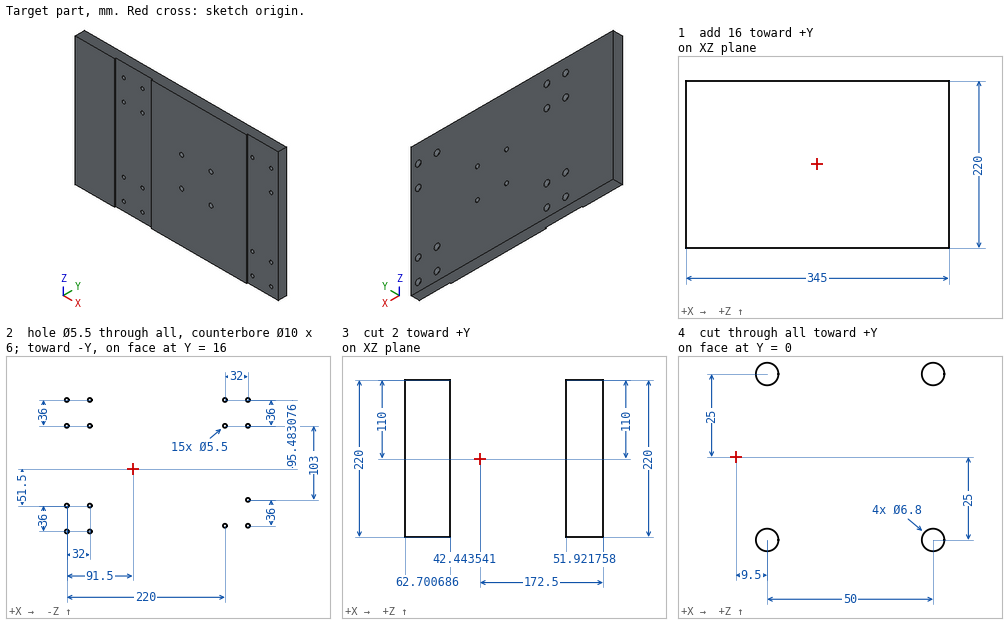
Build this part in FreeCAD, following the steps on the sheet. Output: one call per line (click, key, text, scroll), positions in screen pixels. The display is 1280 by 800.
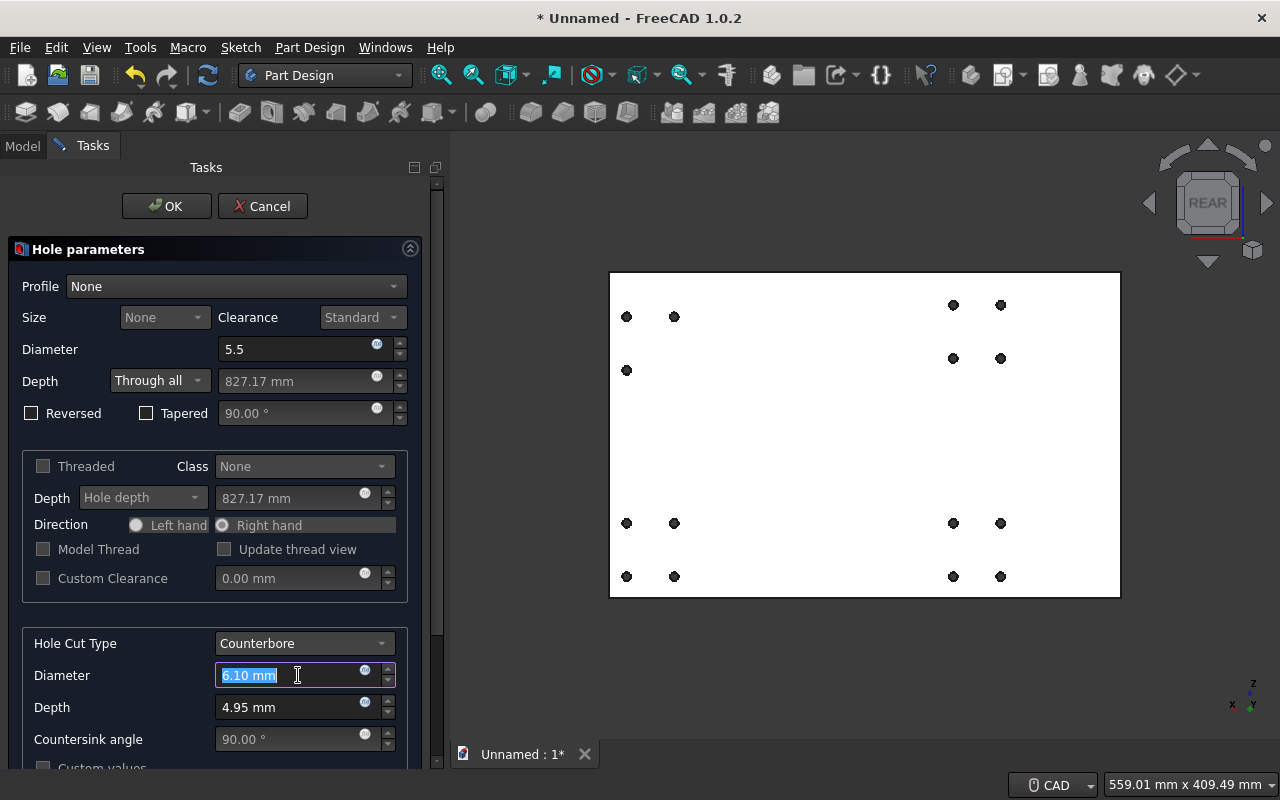
text(10)
key(Tab)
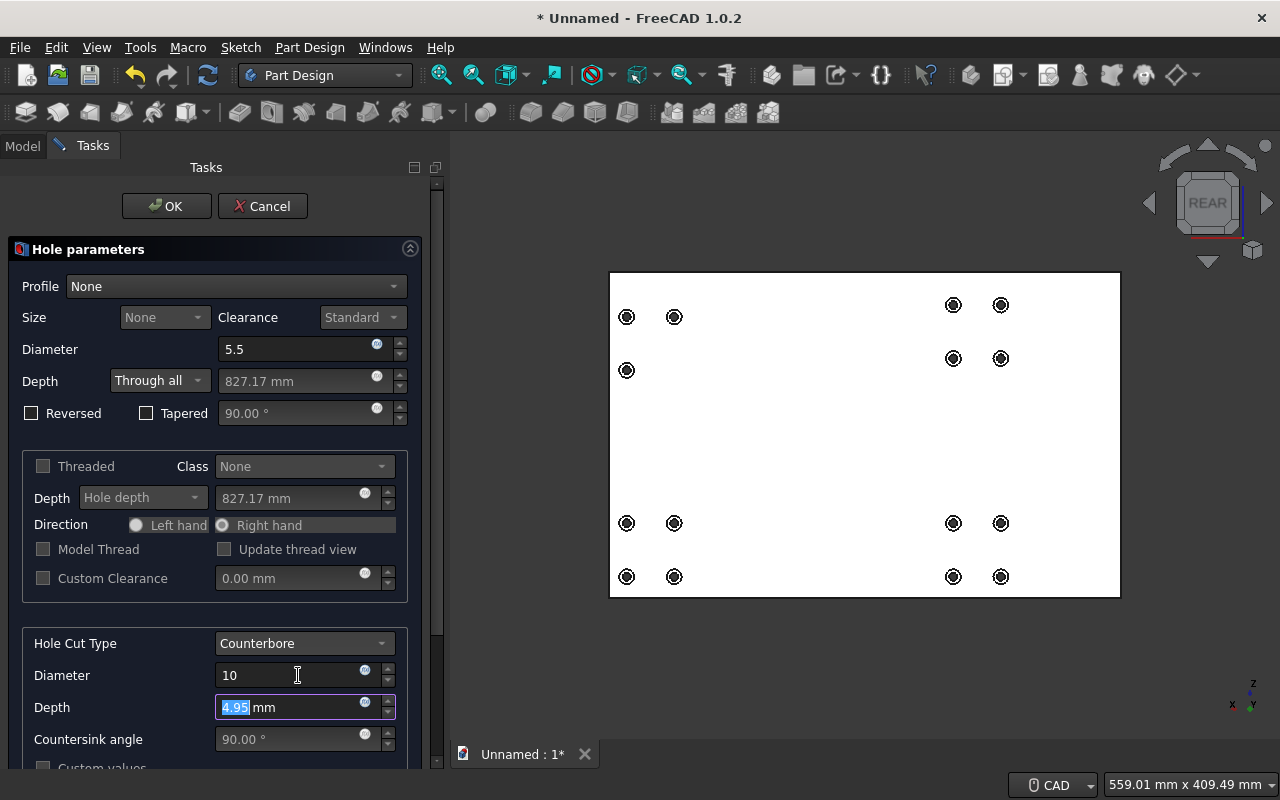
text(6)
key(Tab)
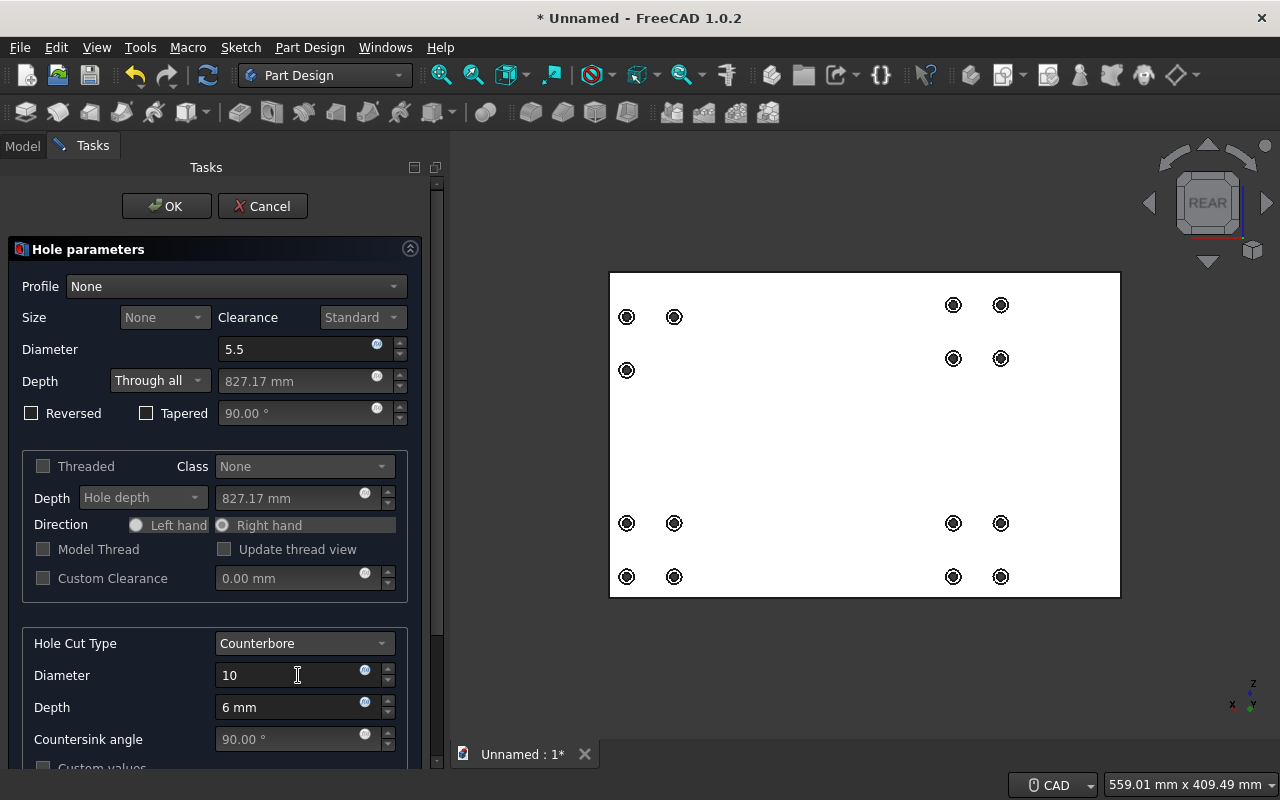
click(167, 206)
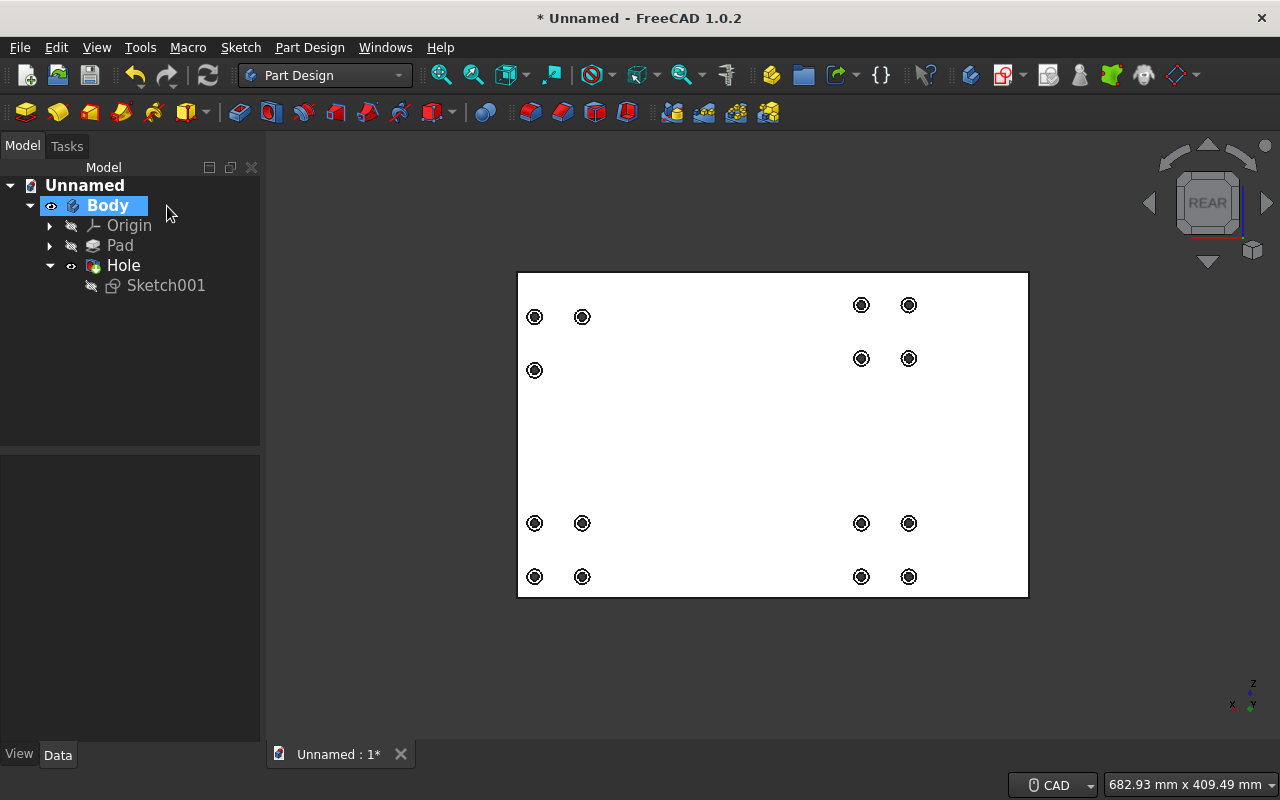
click(1004, 76)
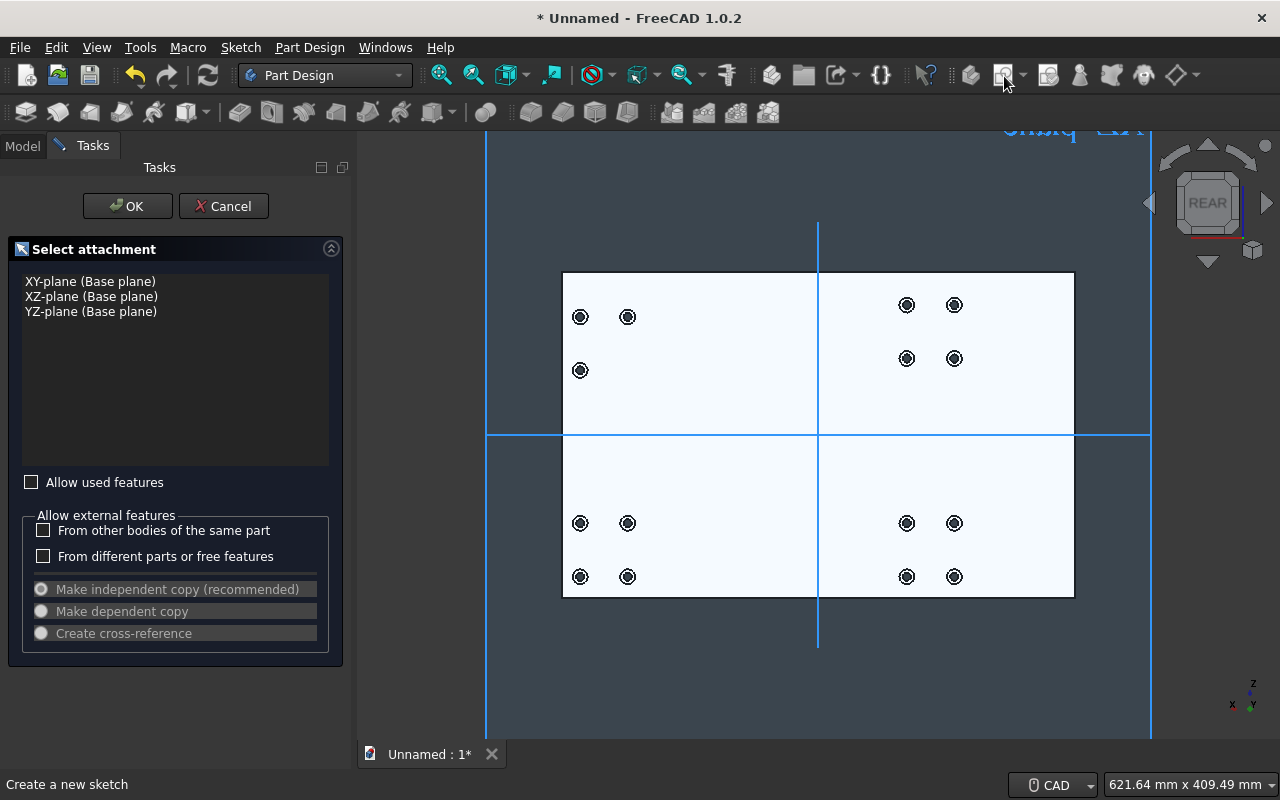
click(82, 296)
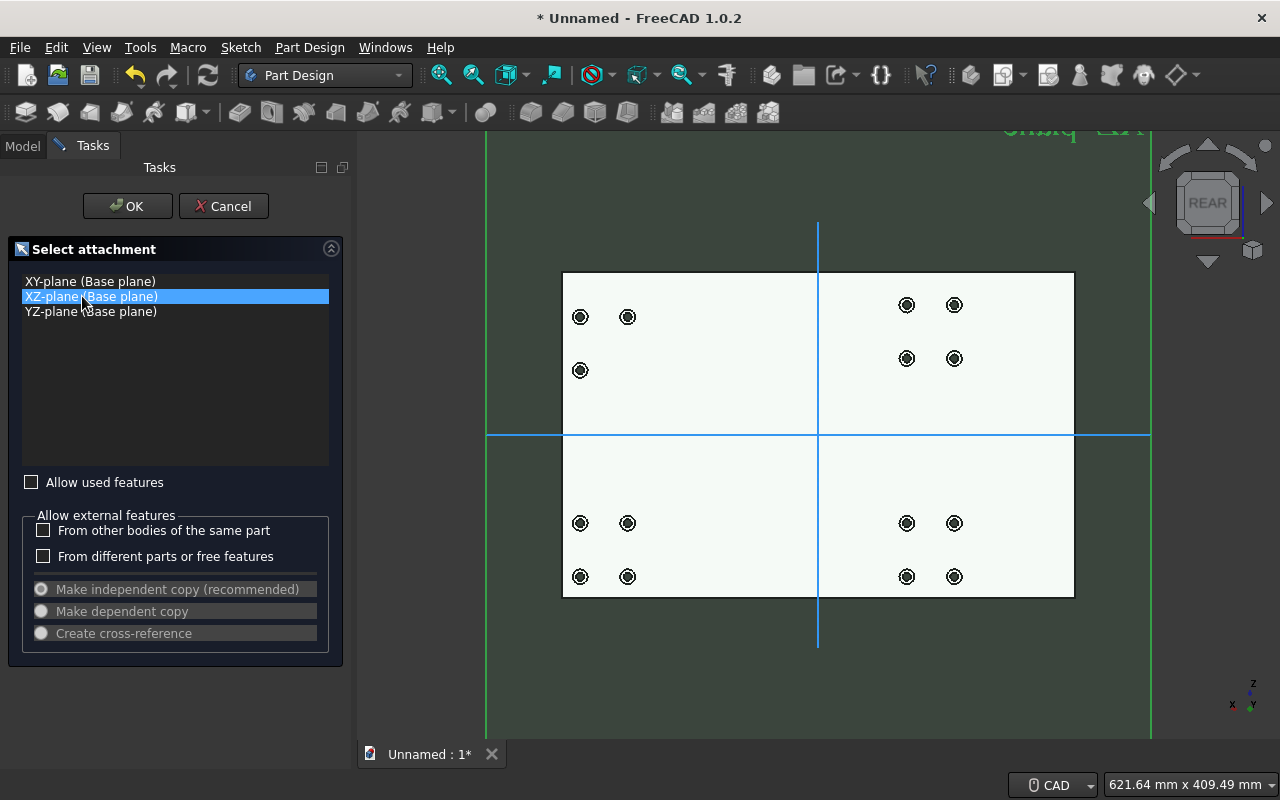
click(128, 206)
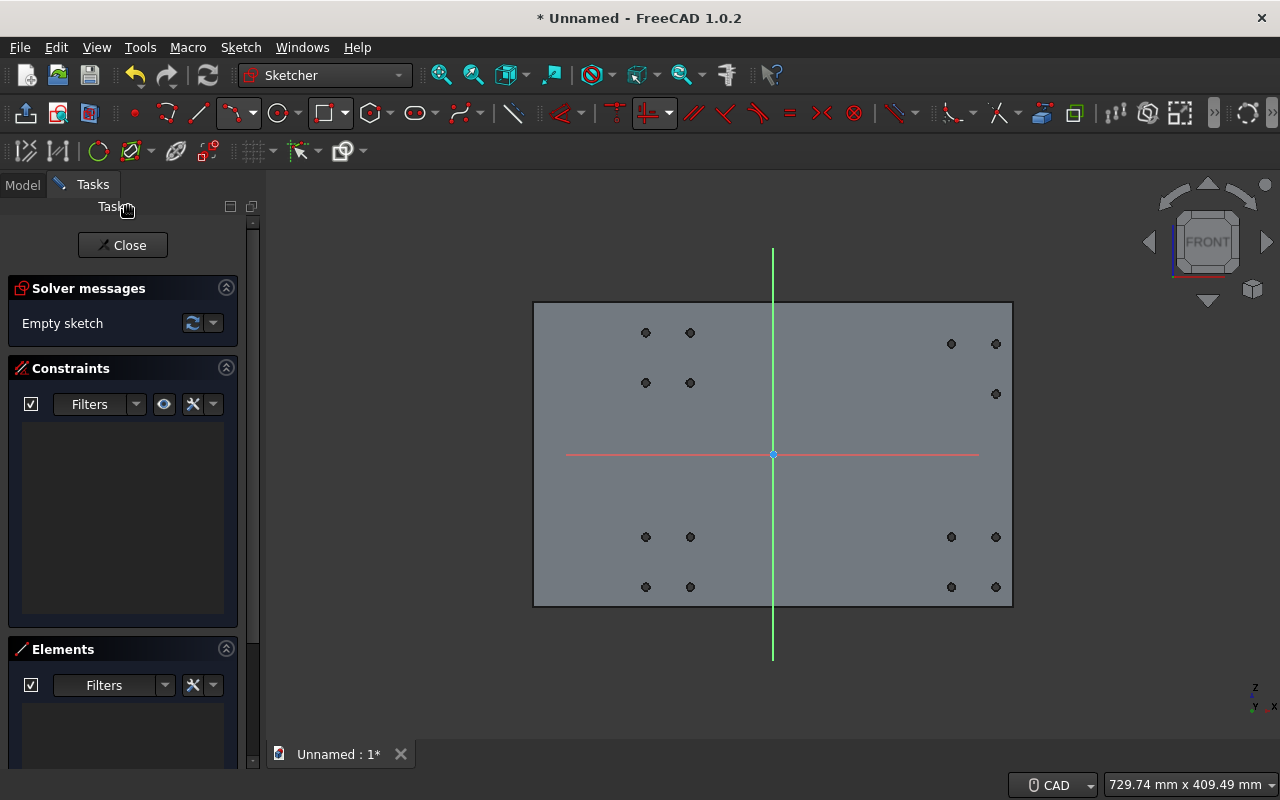
click(324, 114)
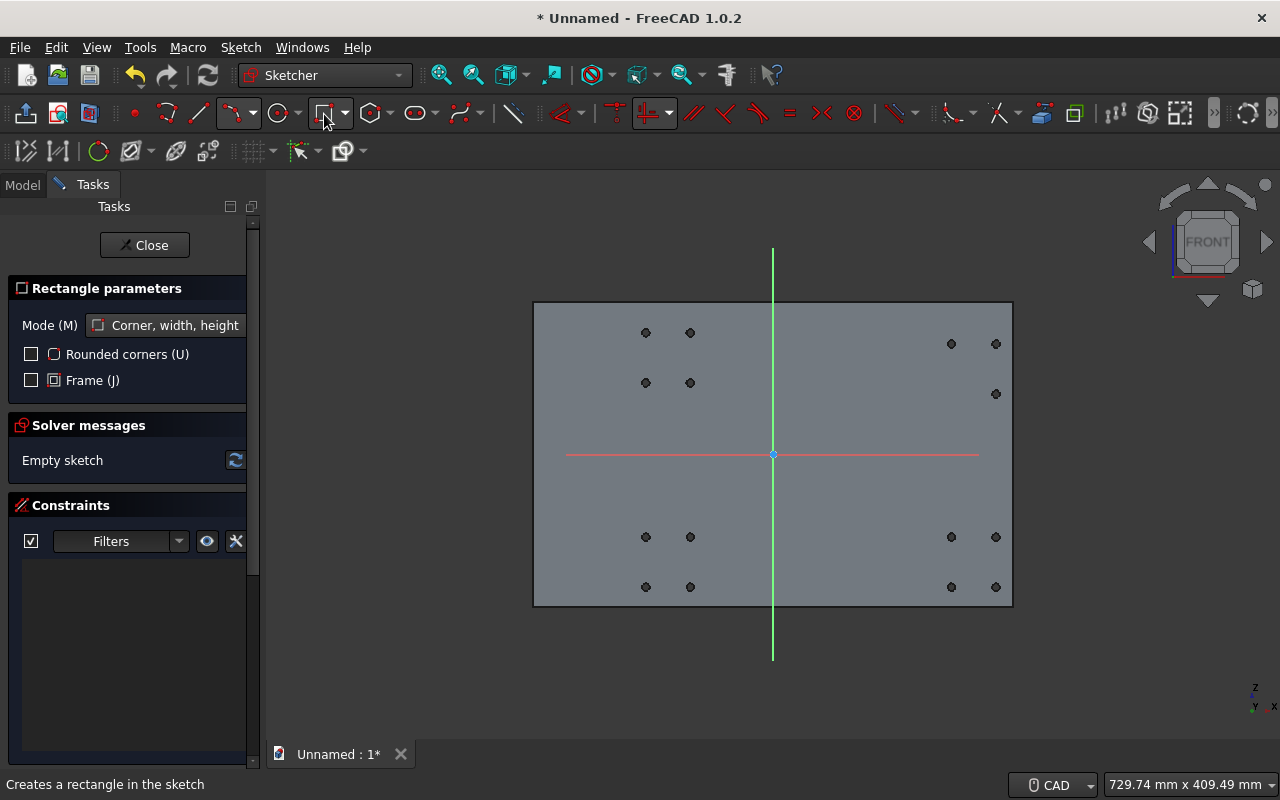
click(627, 302)
move(714, 607)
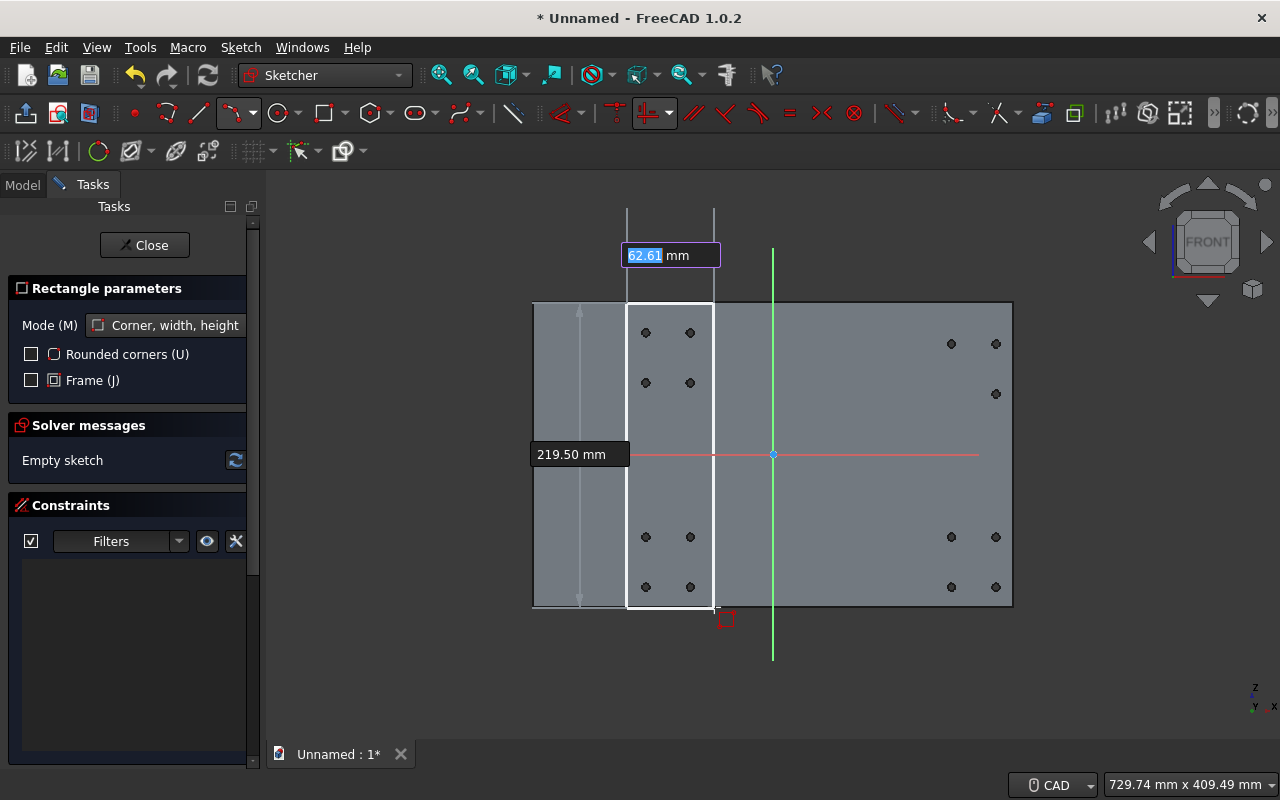
text(62.700686)
key(Tab)
text(220)
key(Return)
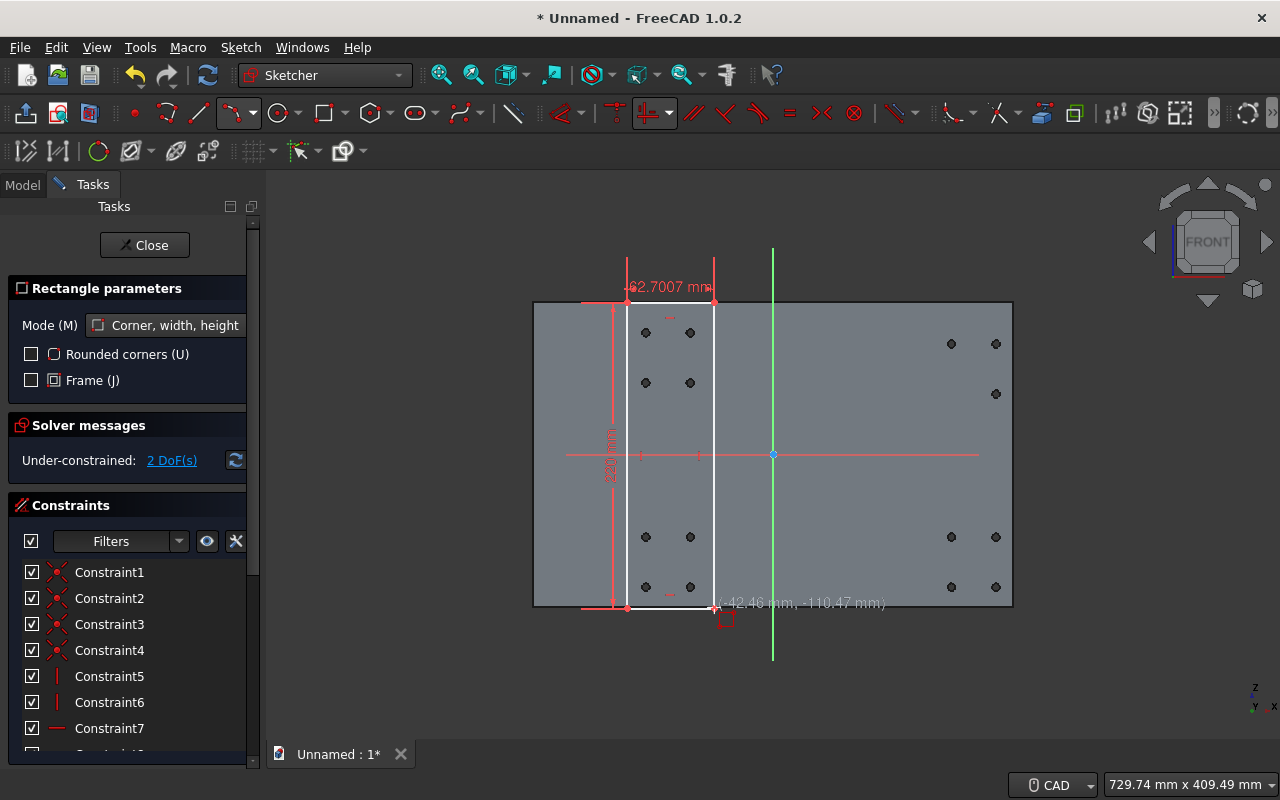
click(941, 302)
move(1013, 607)